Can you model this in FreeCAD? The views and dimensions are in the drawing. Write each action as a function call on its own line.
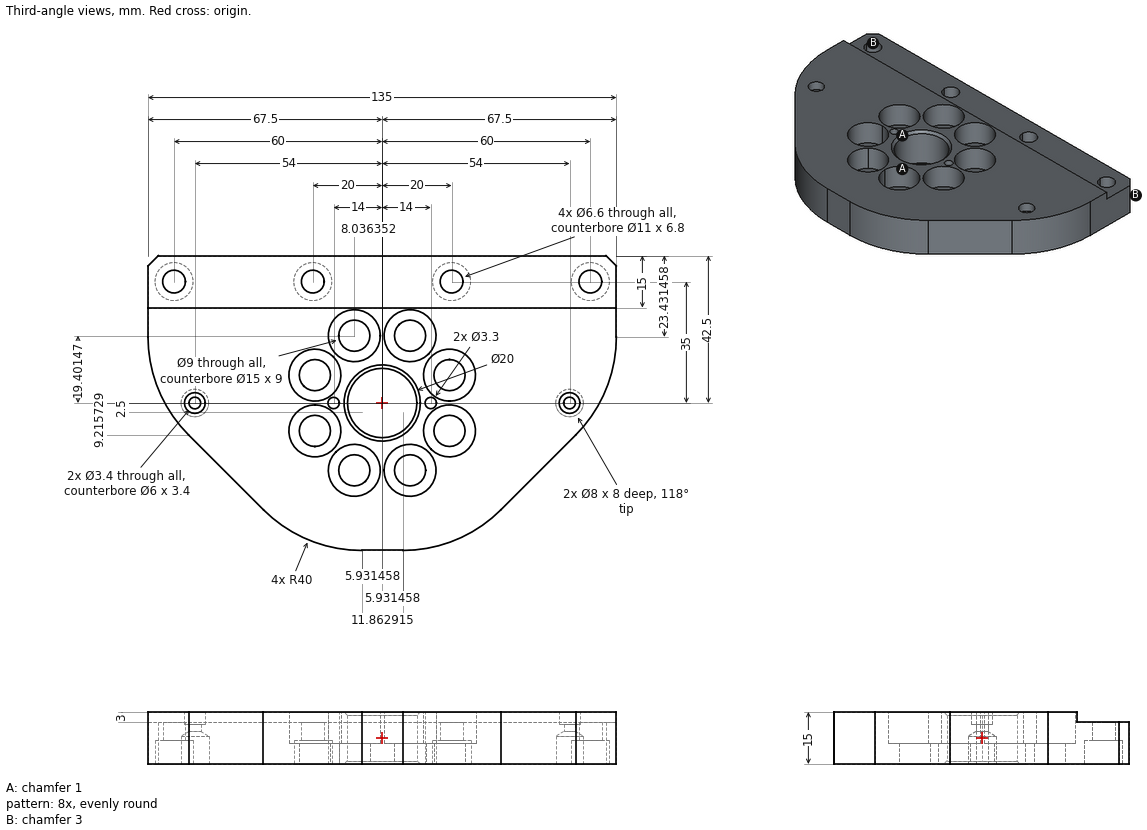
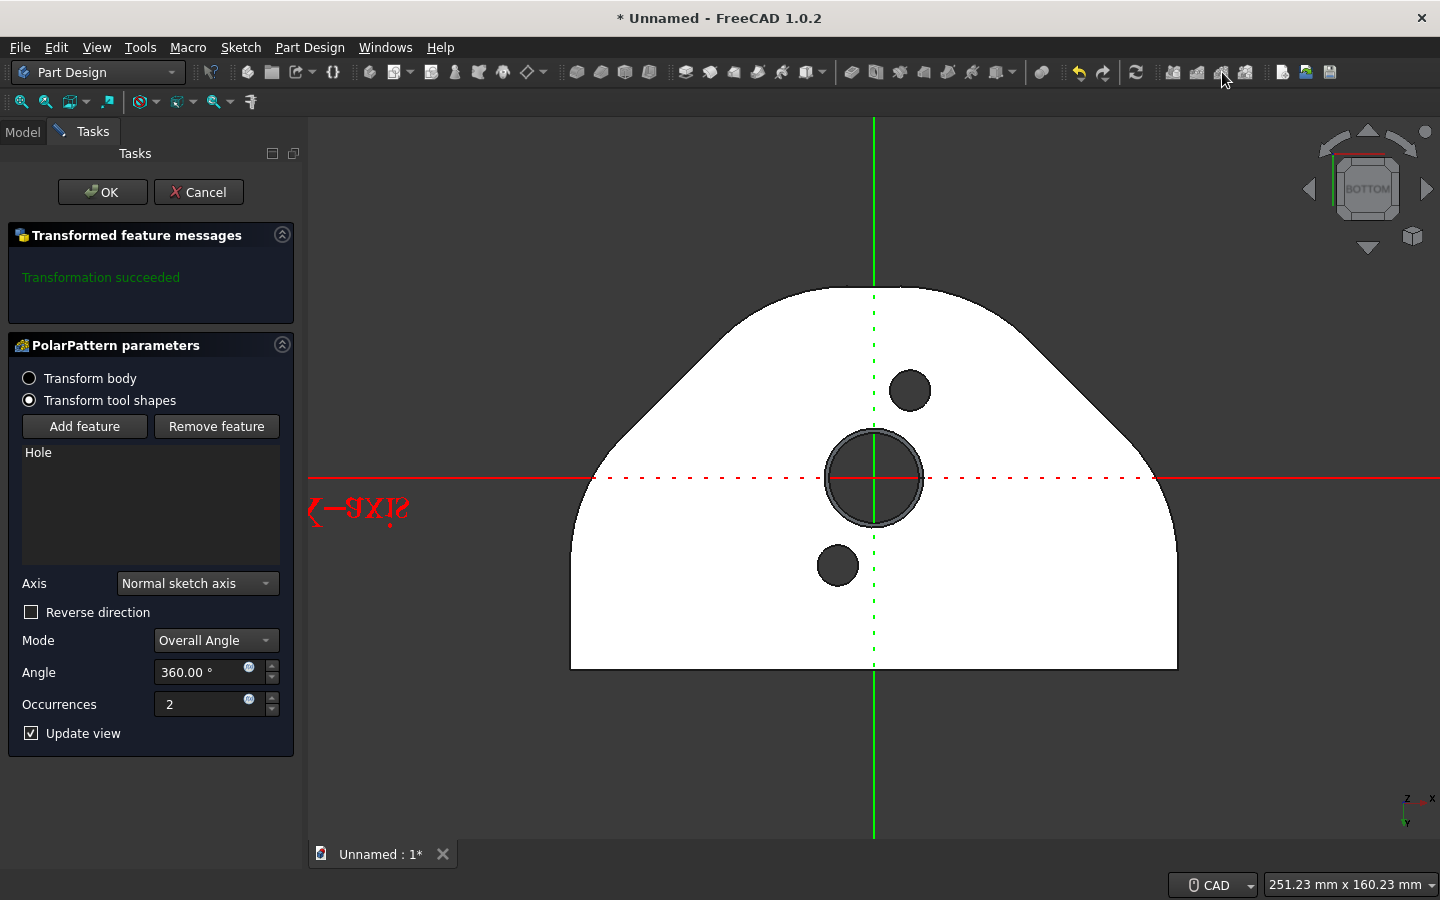
click(198, 584)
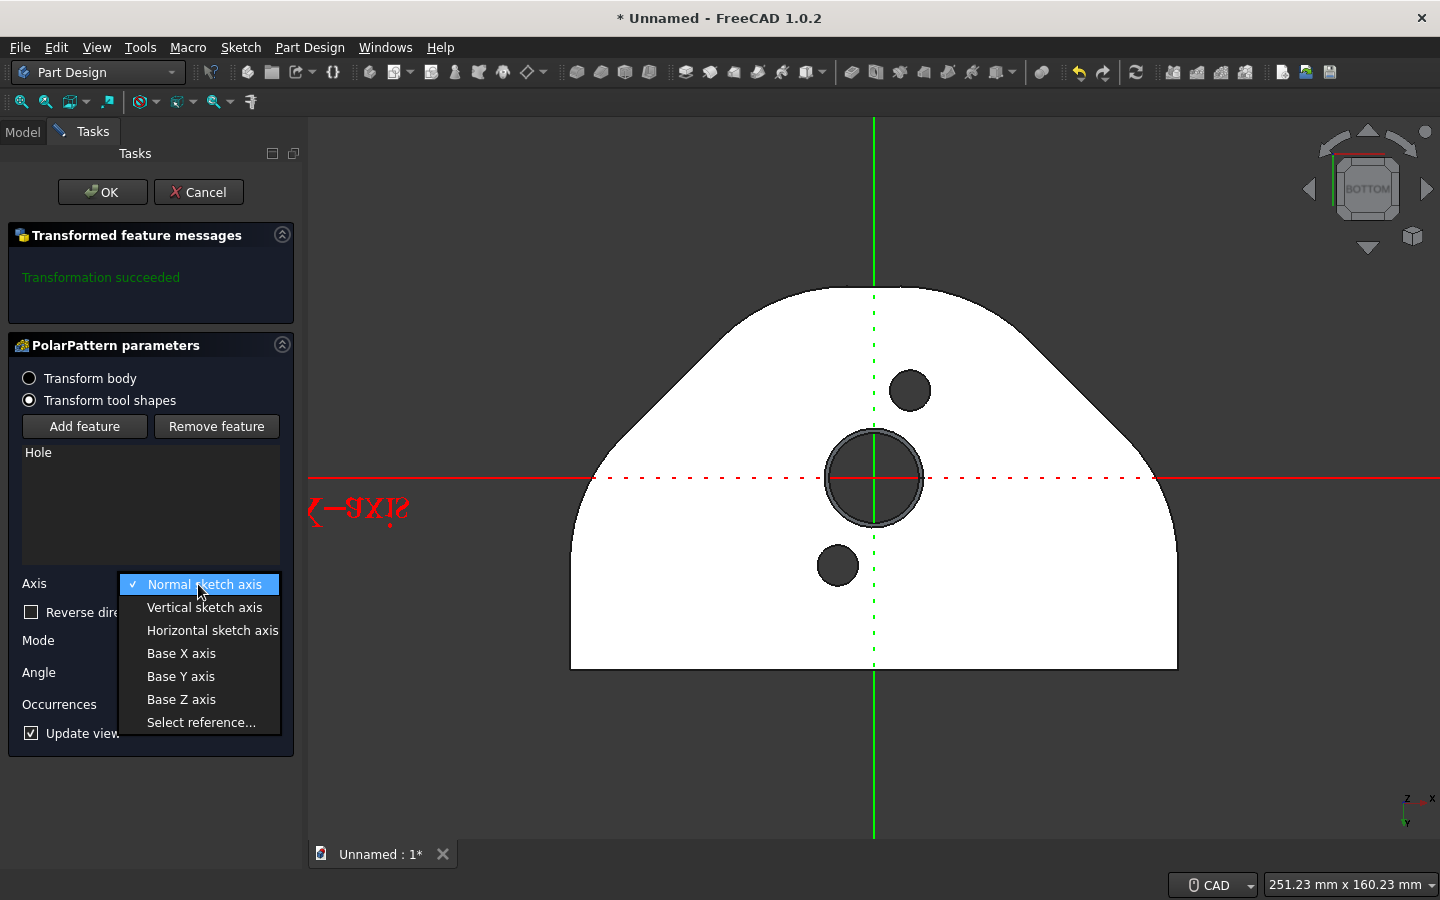
click(198, 700)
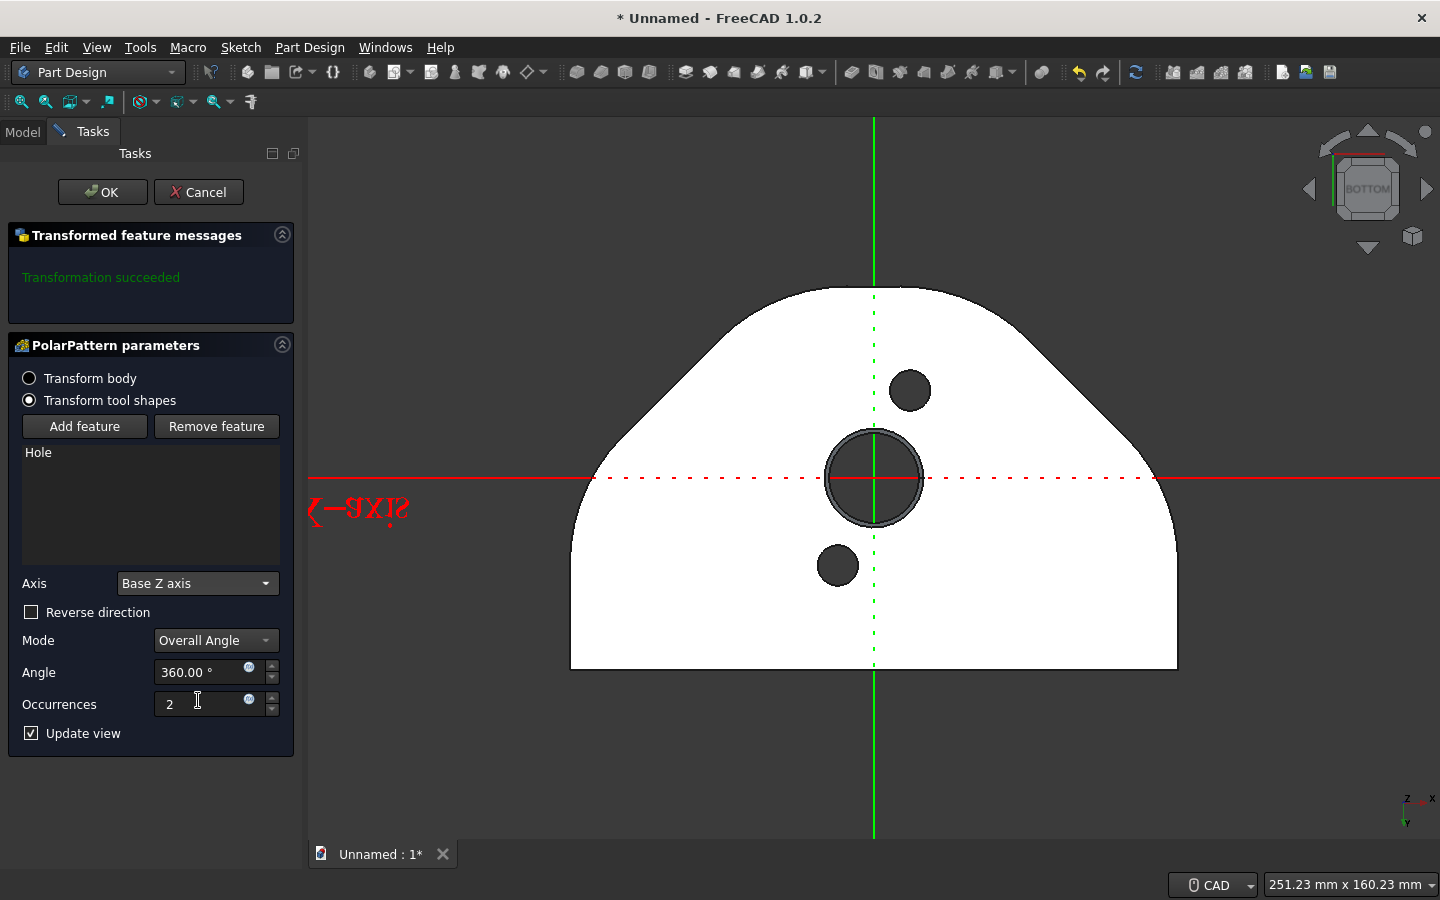
triple_click(209, 704)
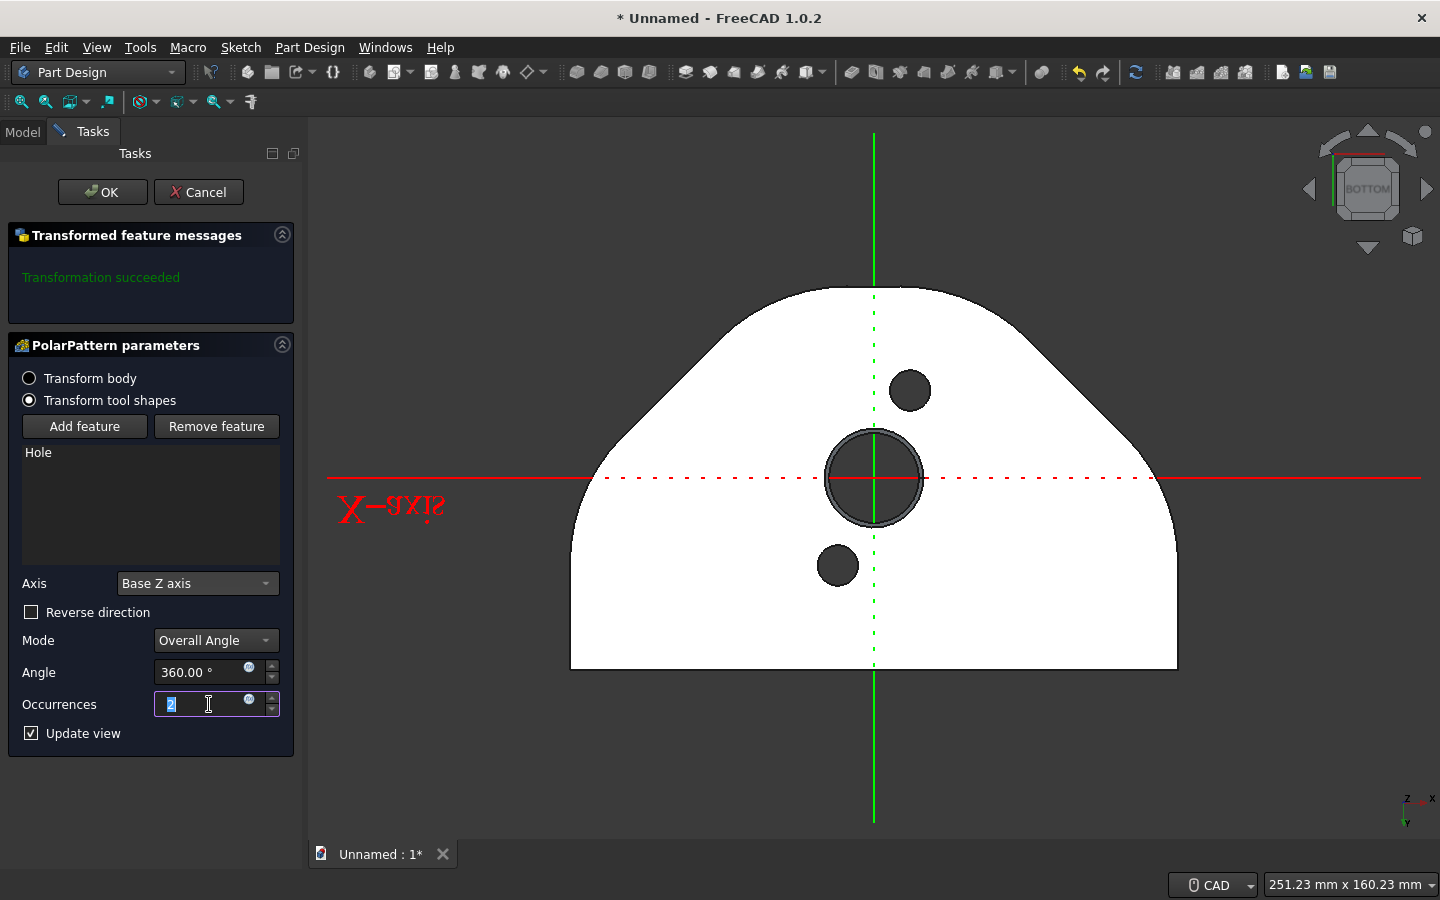
text(8)
key(Tab)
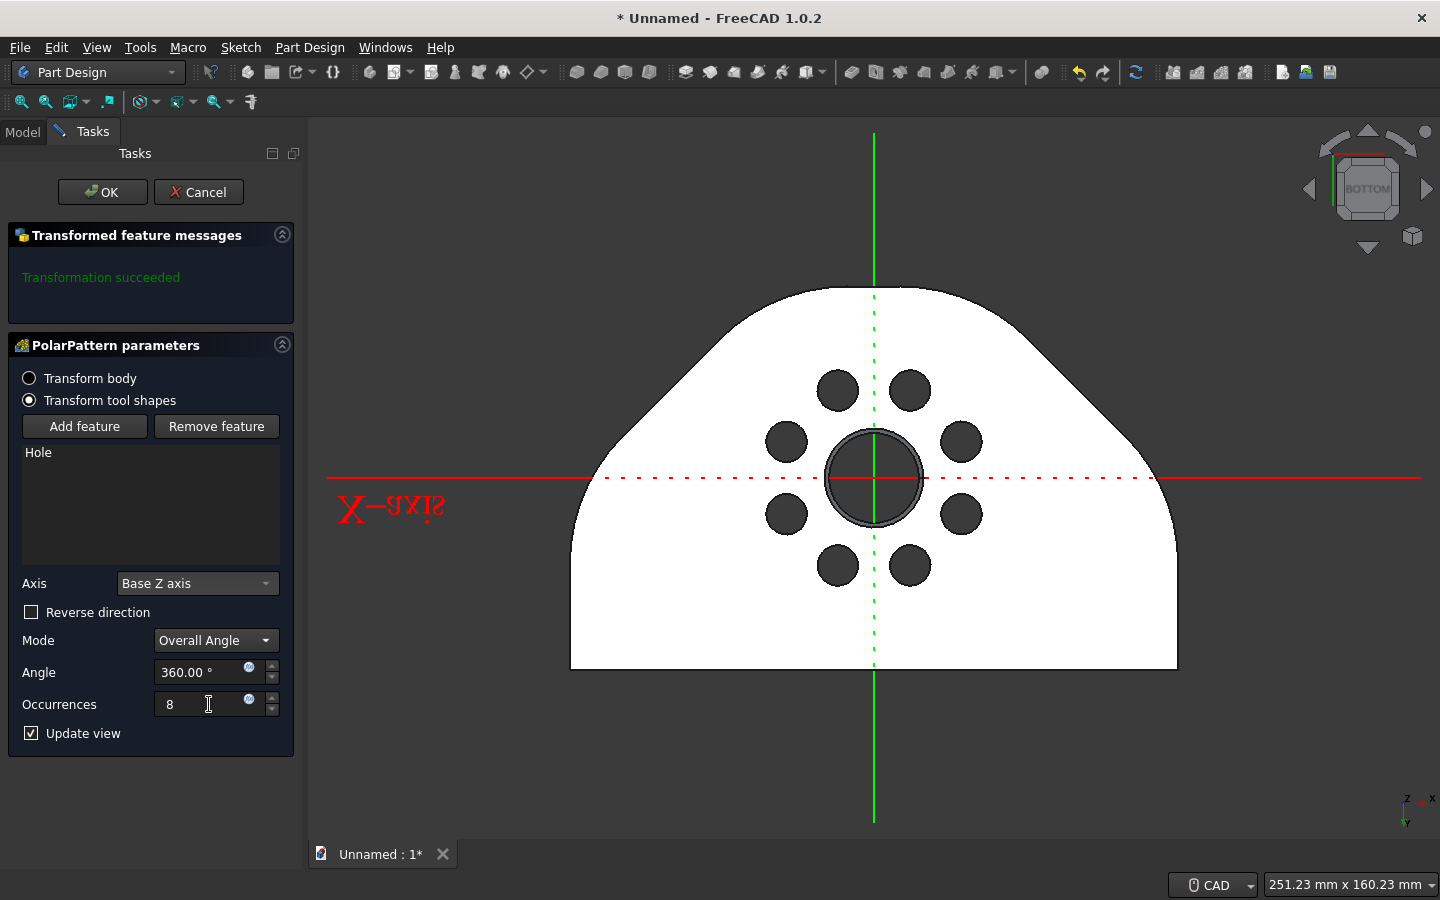
click(103, 192)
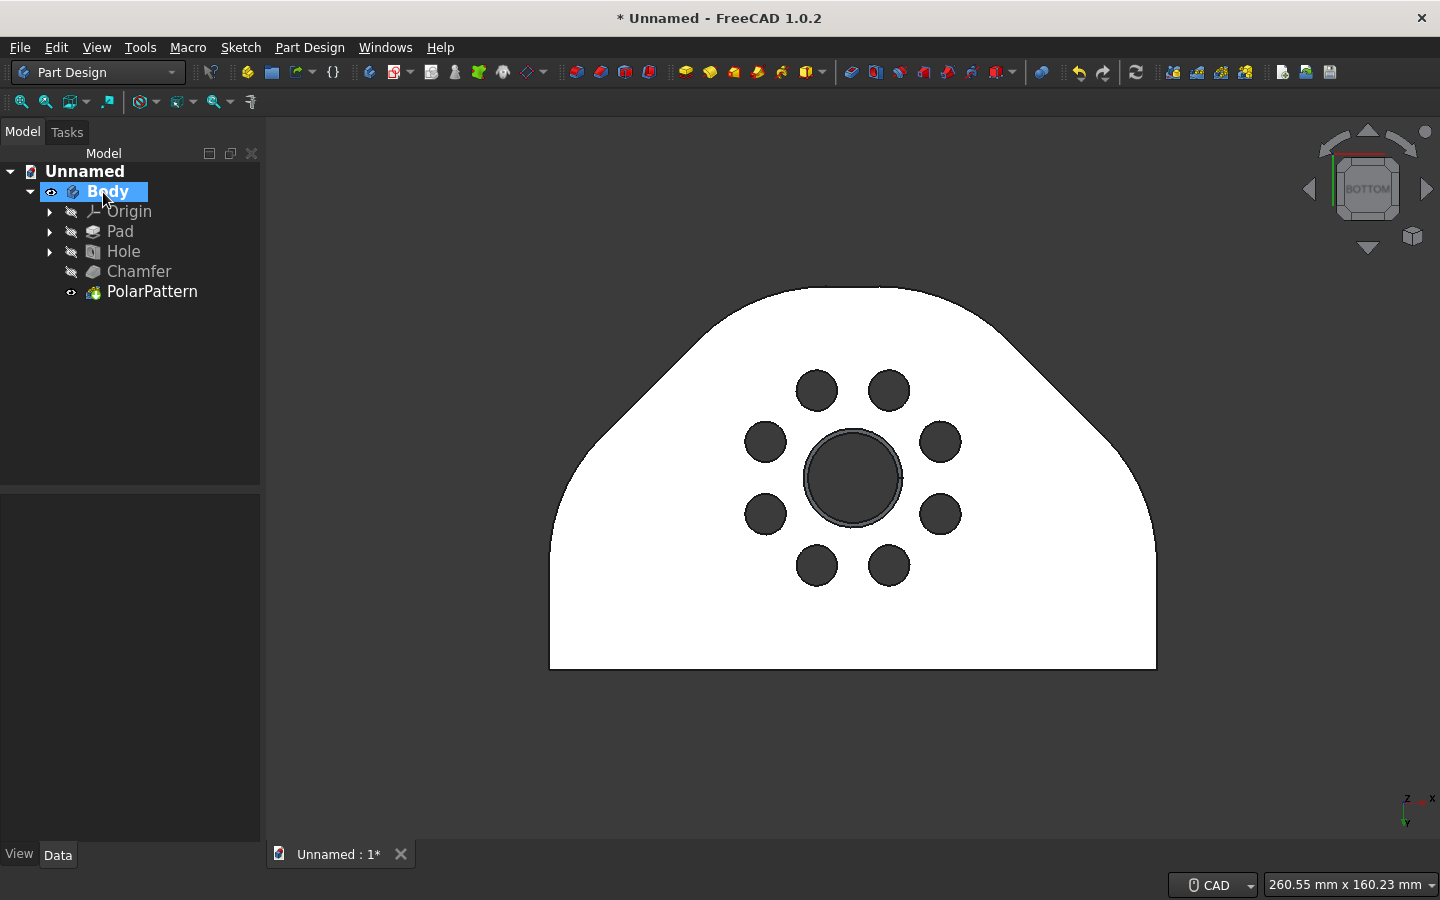
key(0)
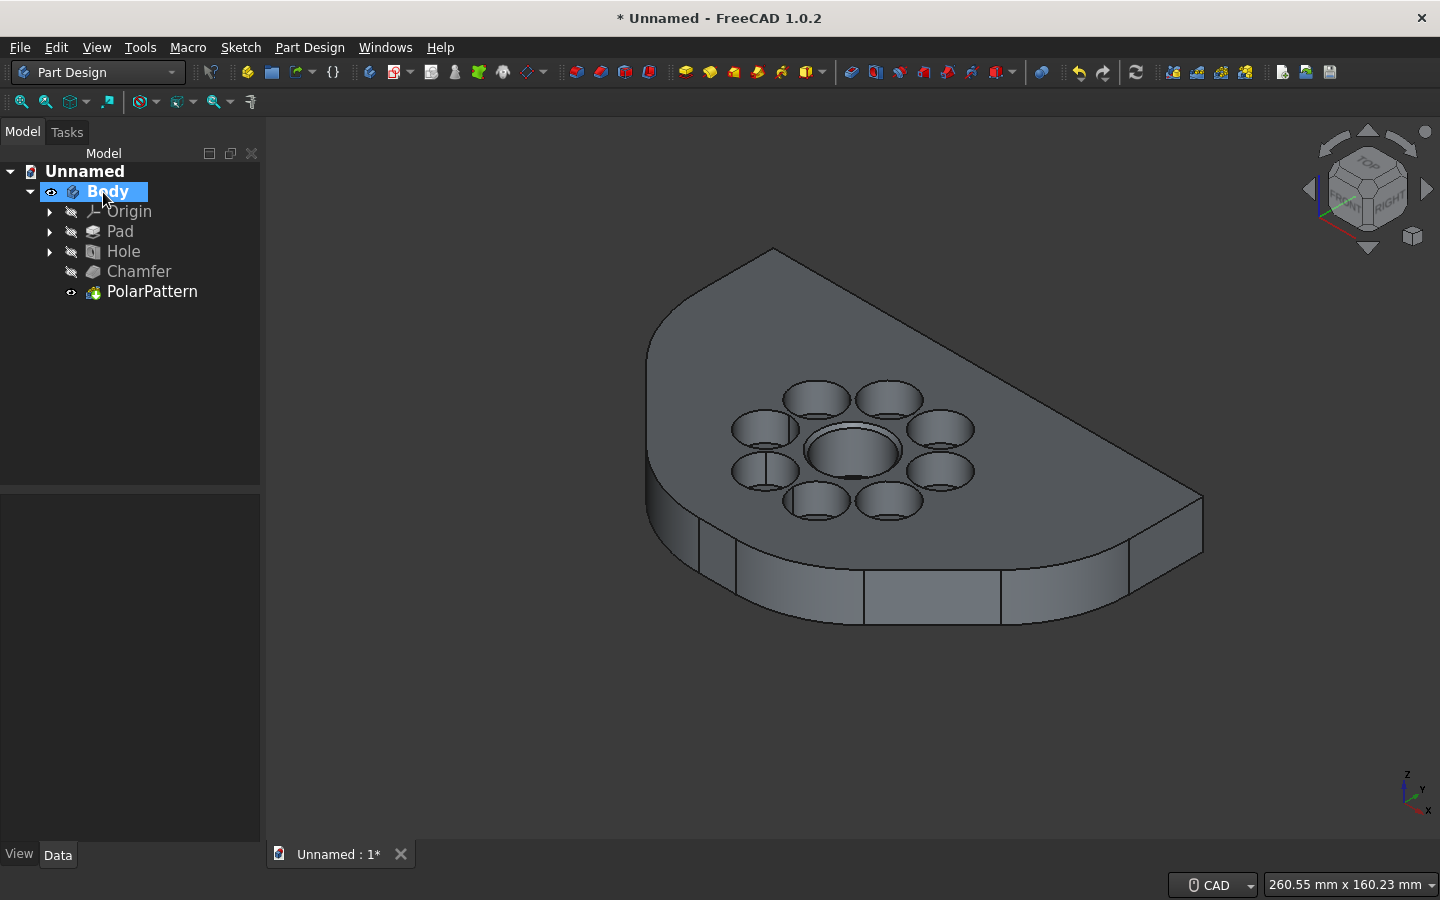
click(1053, 476)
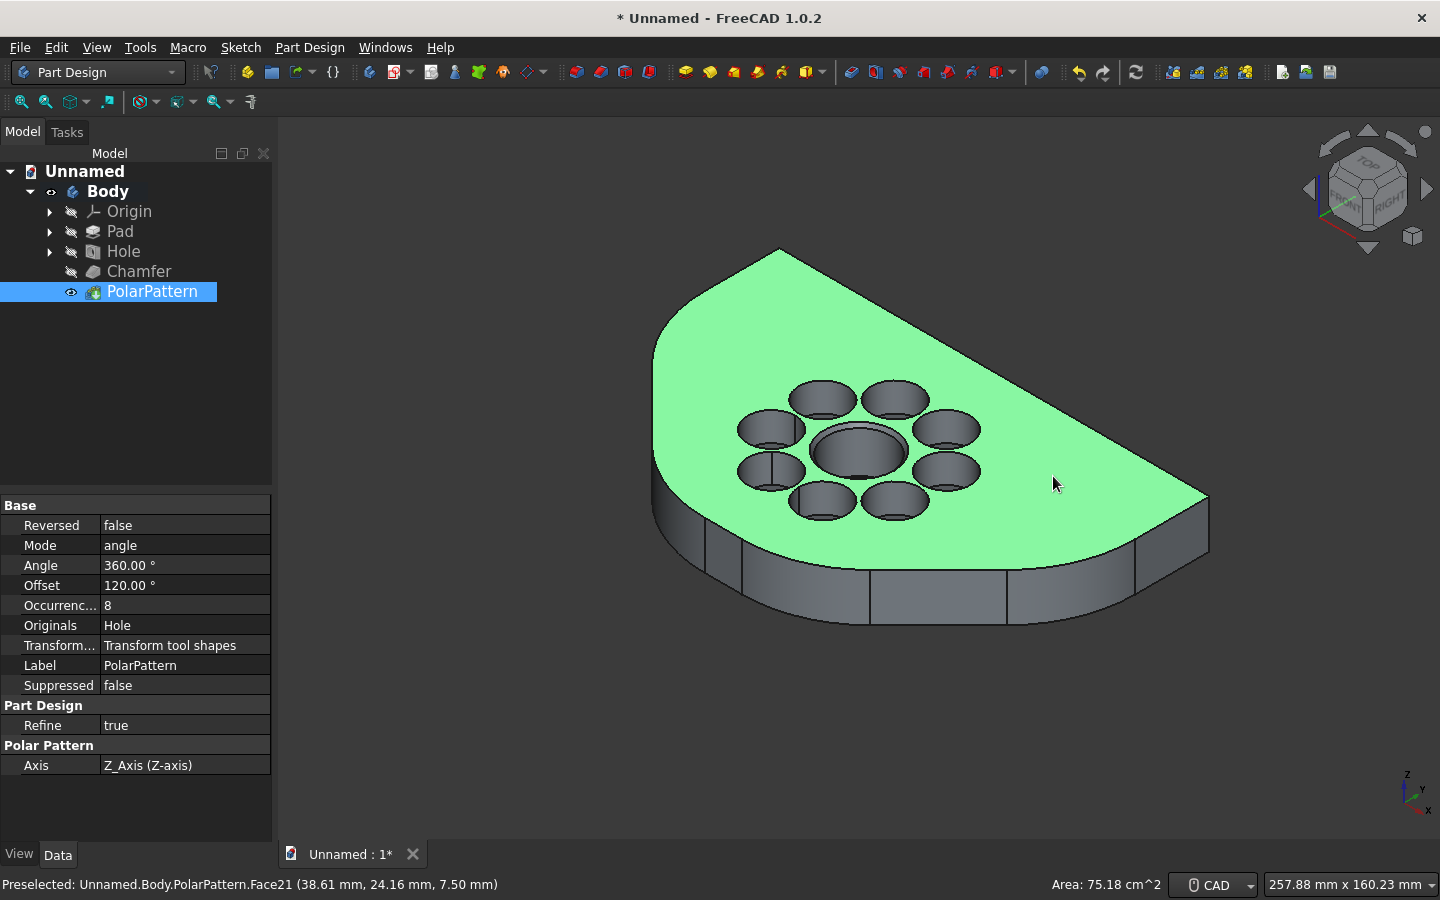
click(394, 72)